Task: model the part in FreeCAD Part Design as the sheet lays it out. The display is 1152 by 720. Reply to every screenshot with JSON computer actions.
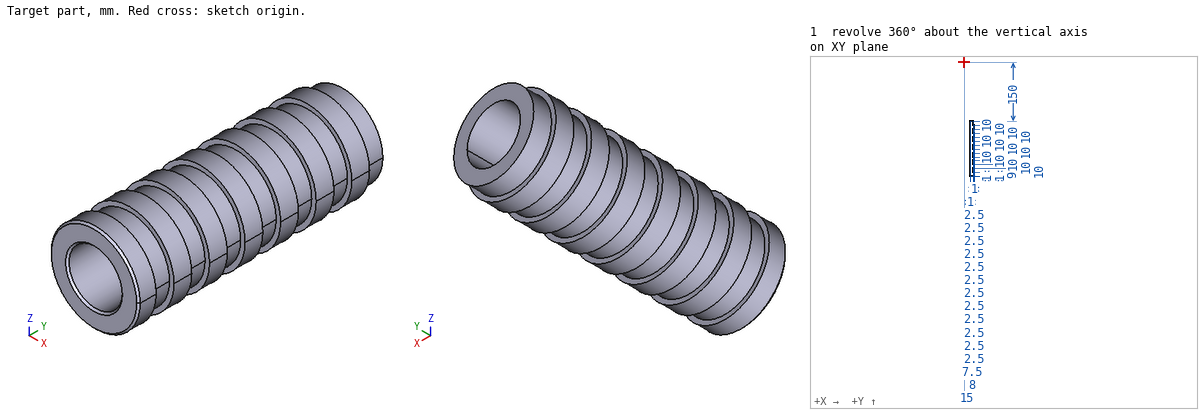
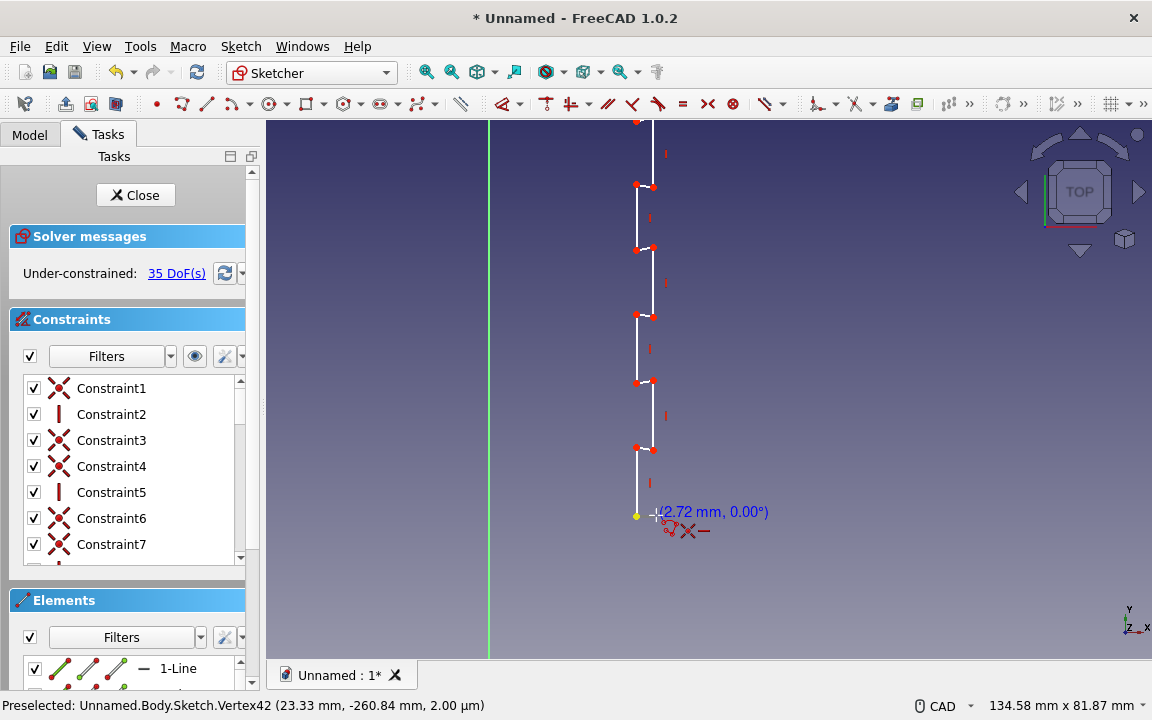
{"action": "left_click", "coordinate": [653, 513]}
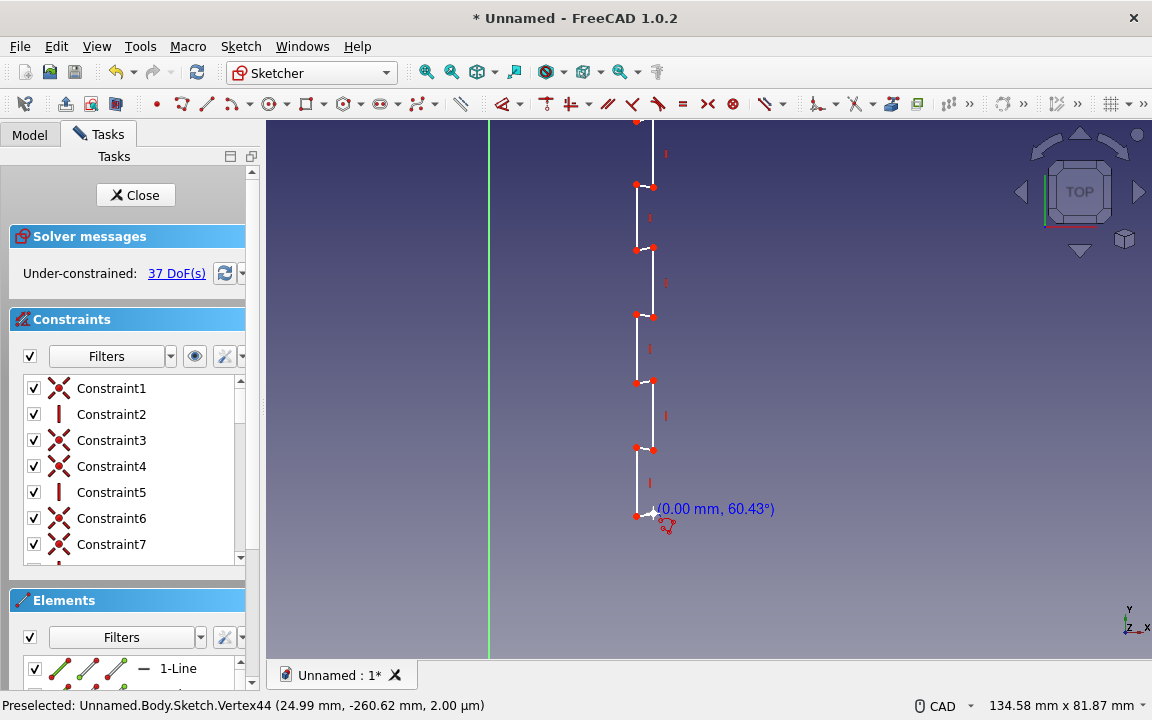
{"action": "scroll", "coordinate": [654, 515], "scroll_direction": "down", "scroll_amount": 9}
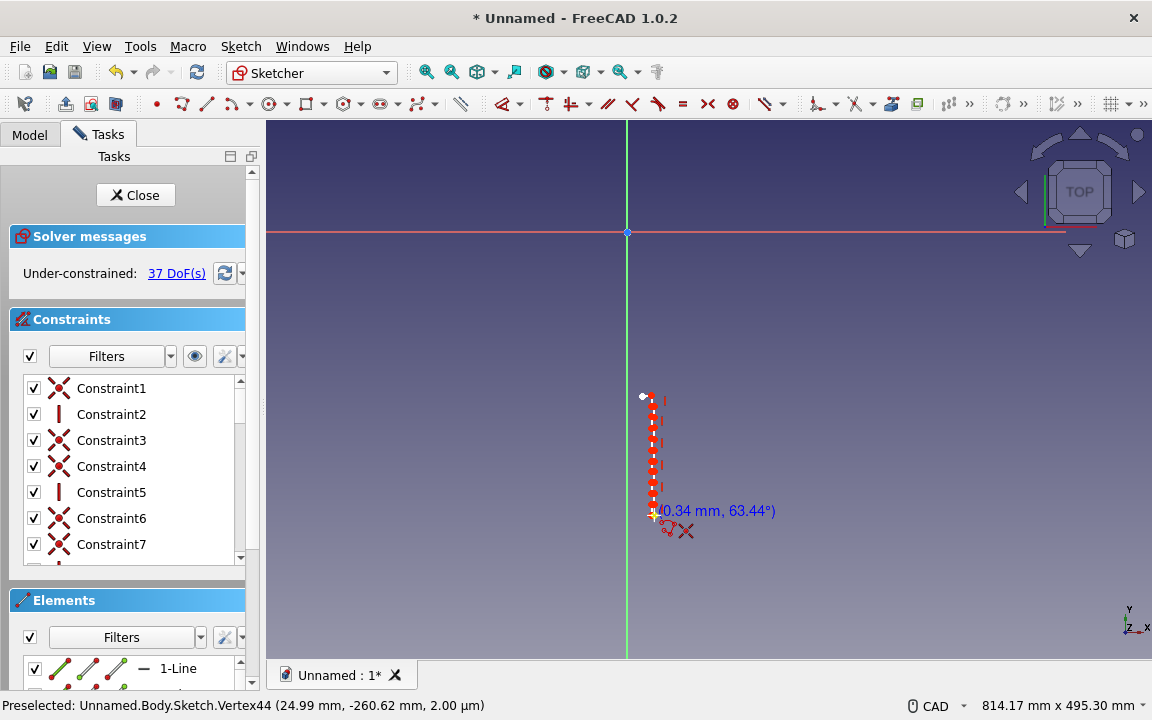
{"action": "scroll", "coordinate": [654, 526], "scroll_direction": "up", "scroll_amount": 2}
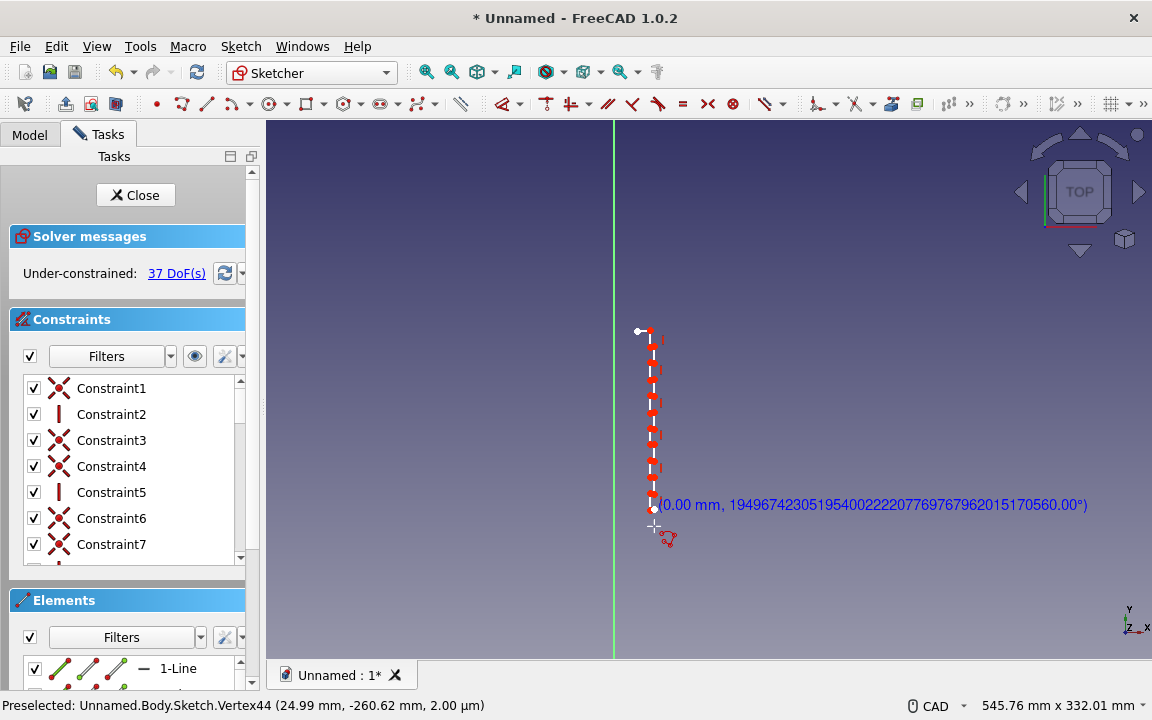
{"action": "left_click", "coordinate": [654, 525]}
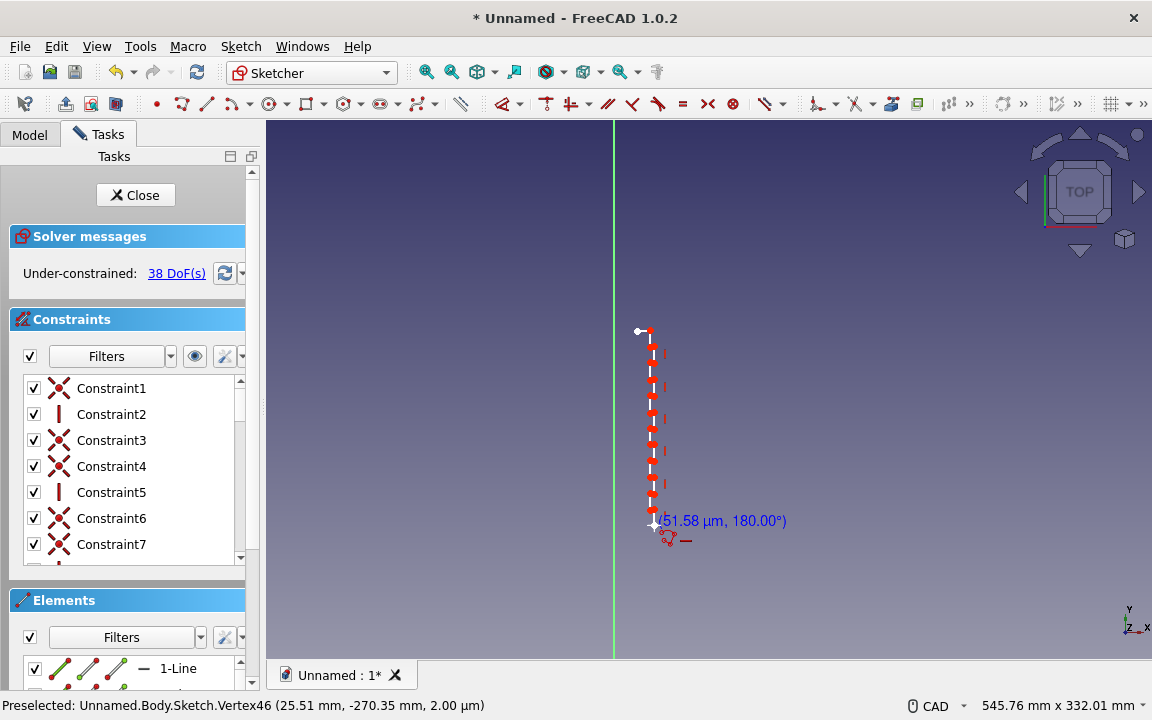
{"action": "scroll", "coordinate": [650, 525], "scroll_direction": "up", "scroll_amount": 7}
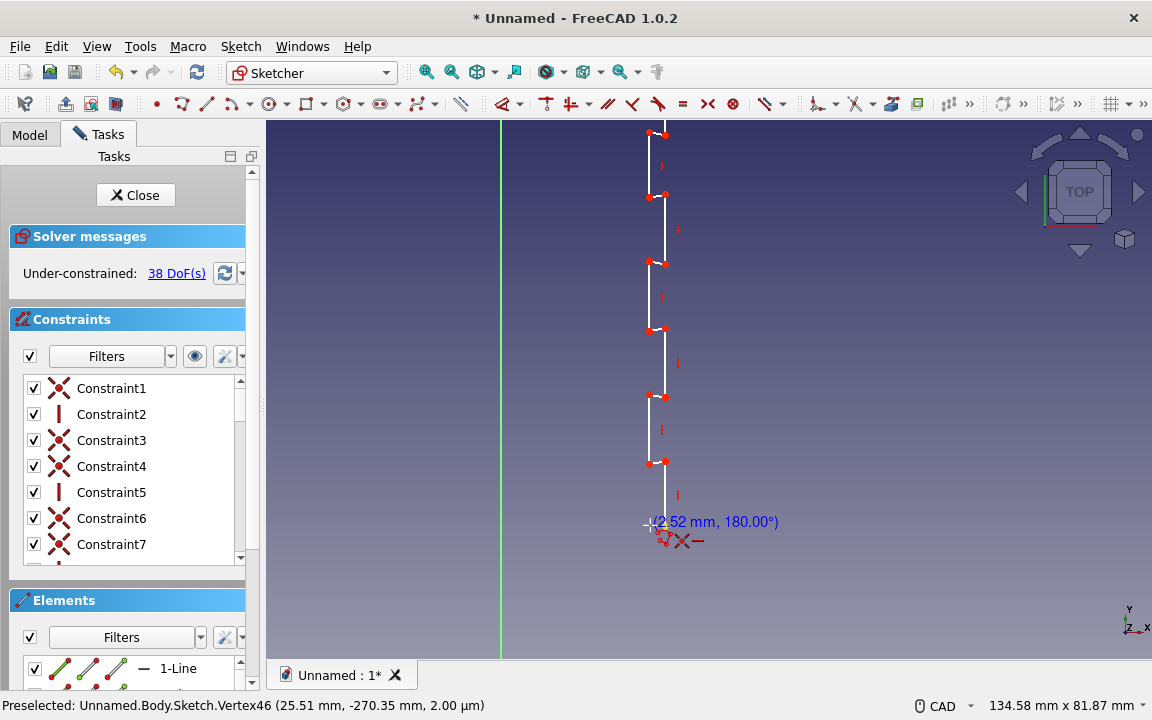
{"action": "left_click", "coordinate": [649, 523]}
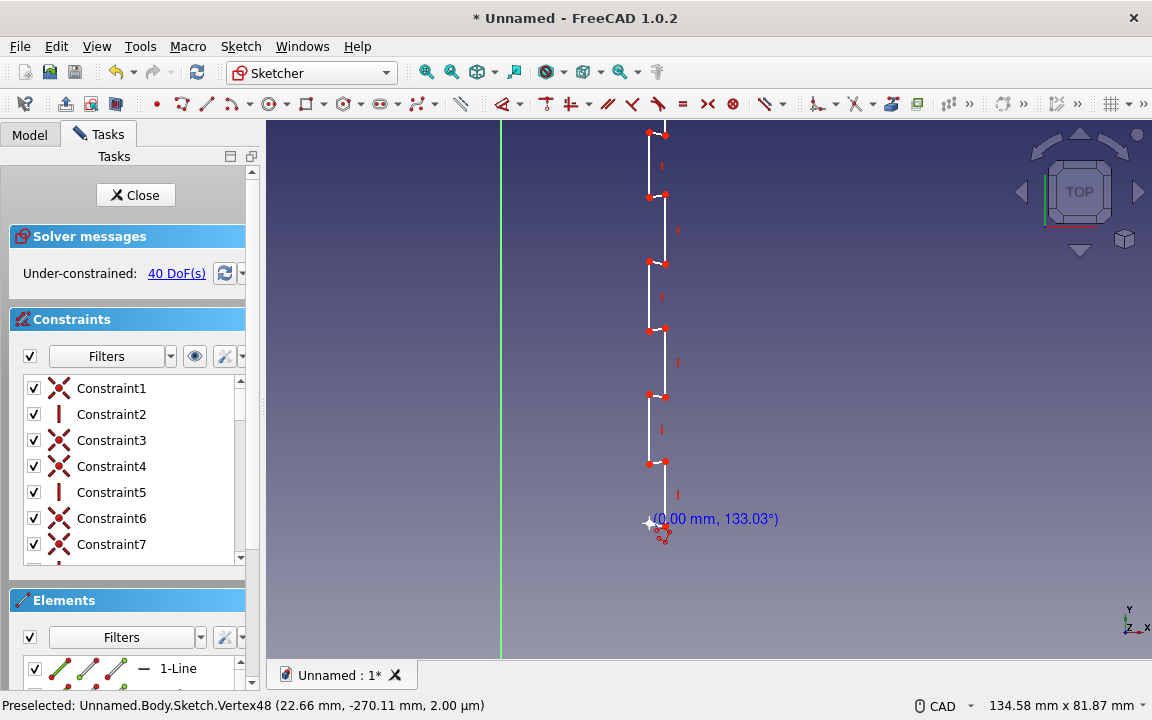
{"action": "scroll", "coordinate": [652, 526], "scroll_direction": "down", "scroll_amount": 9}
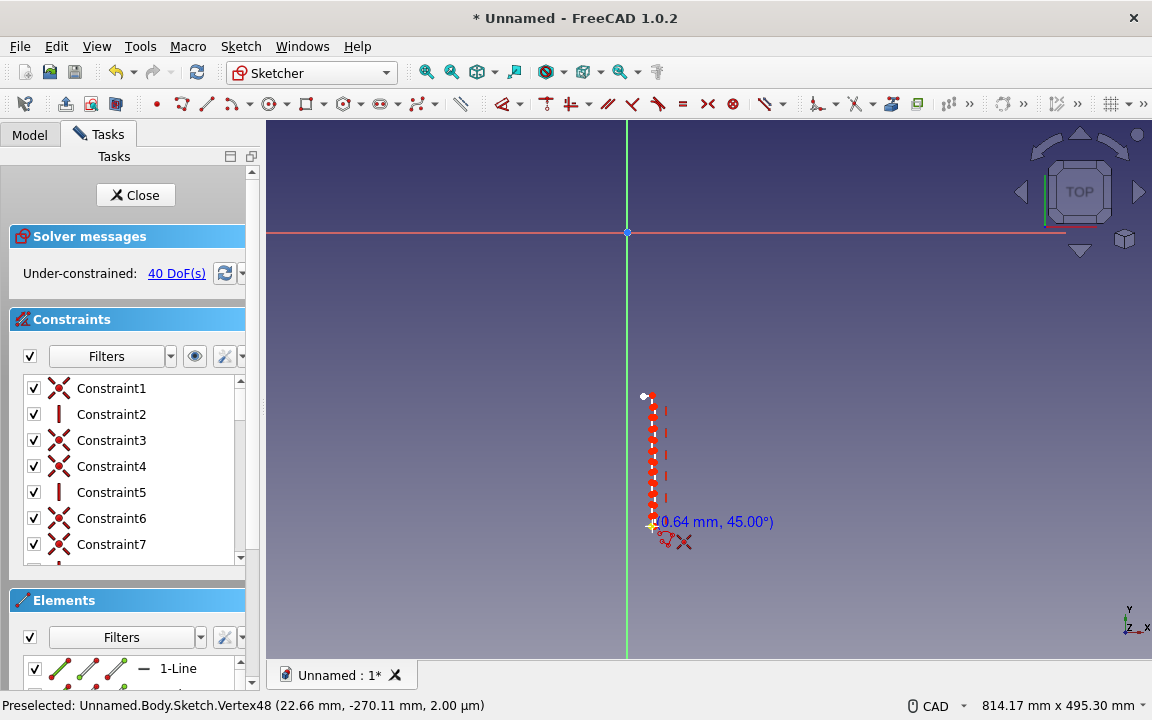
{"action": "scroll", "coordinate": [652, 537], "scroll_direction": "up", "scroll_amount": 2}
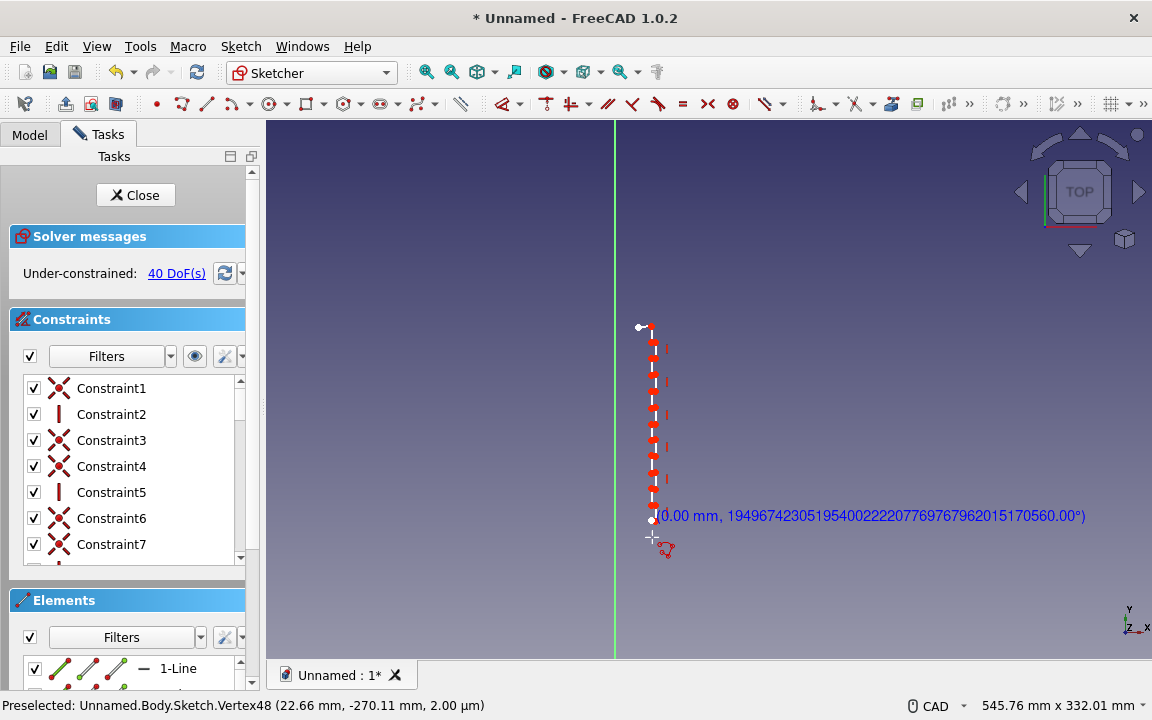
{"action": "left_click", "coordinate": [652, 537]}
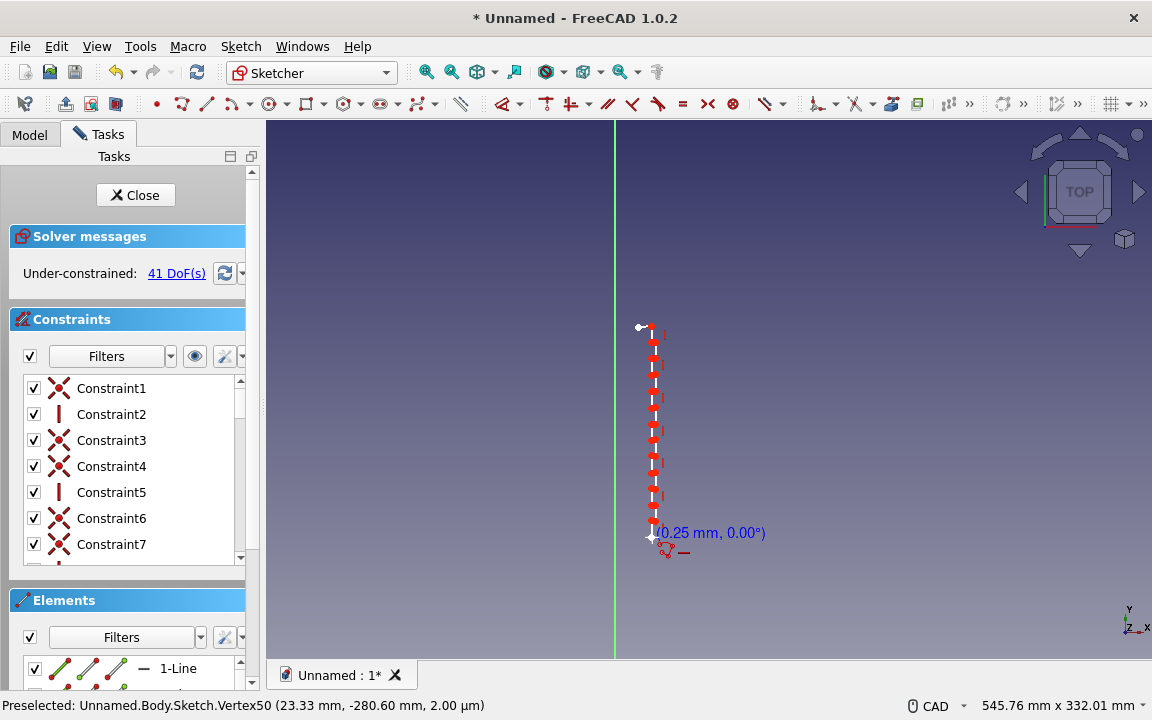
{"action": "scroll", "coordinate": [656, 537], "scroll_direction": "up", "scroll_amount": 7}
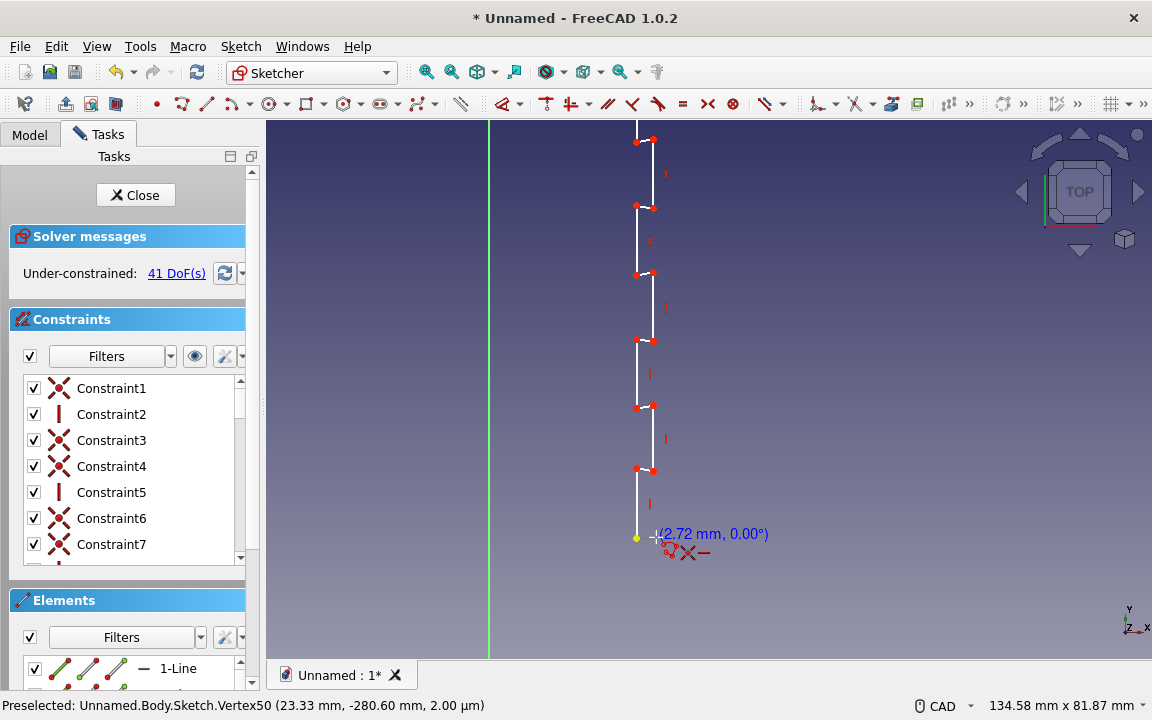
{"action": "left_click", "coordinate": [653, 535]}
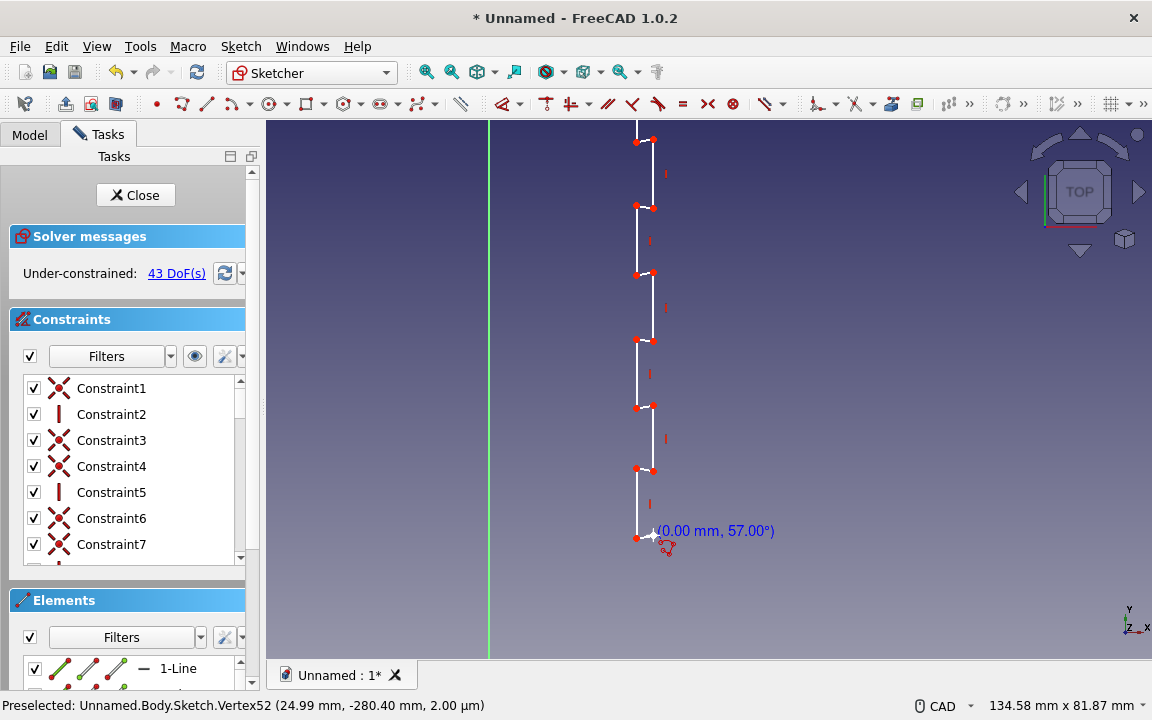
{"action": "scroll", "coordinate": [654, 537], "scroll_direction": "down", "scroll_amount": 9}